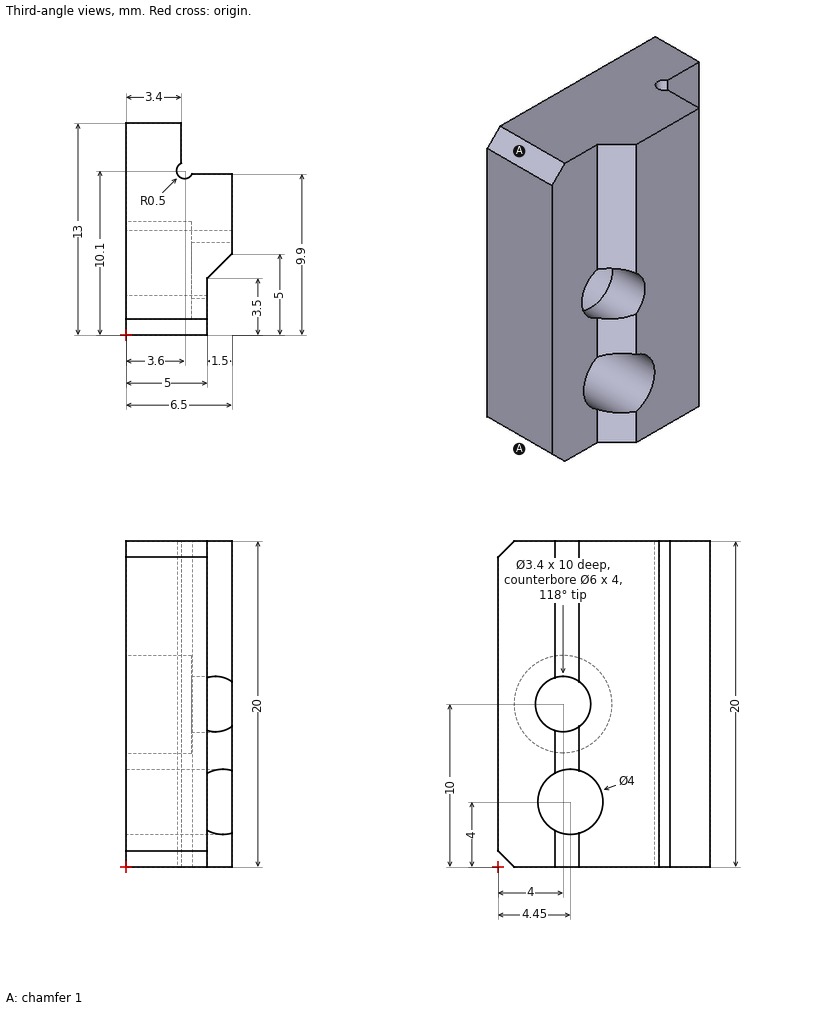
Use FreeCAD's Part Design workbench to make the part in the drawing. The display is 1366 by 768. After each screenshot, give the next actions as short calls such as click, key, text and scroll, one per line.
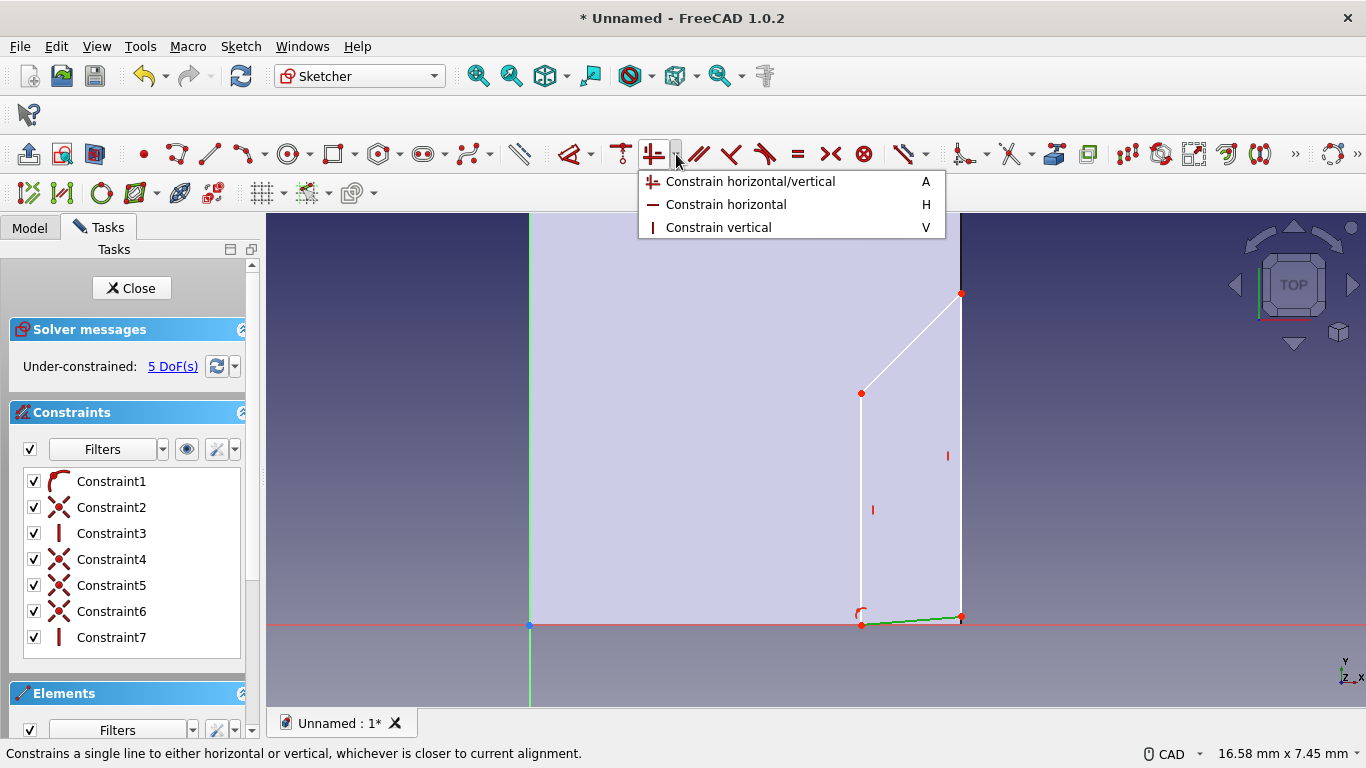
click(792, 204)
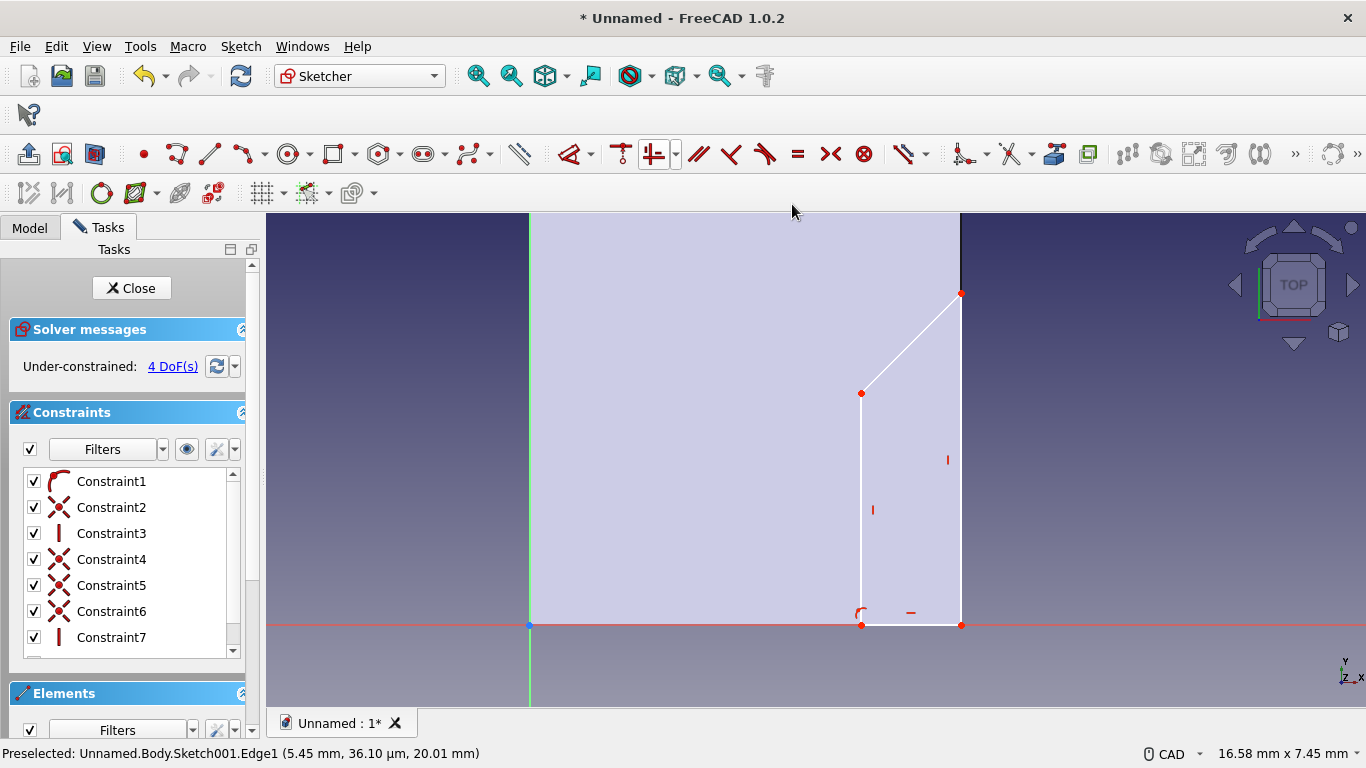
click(568, 154)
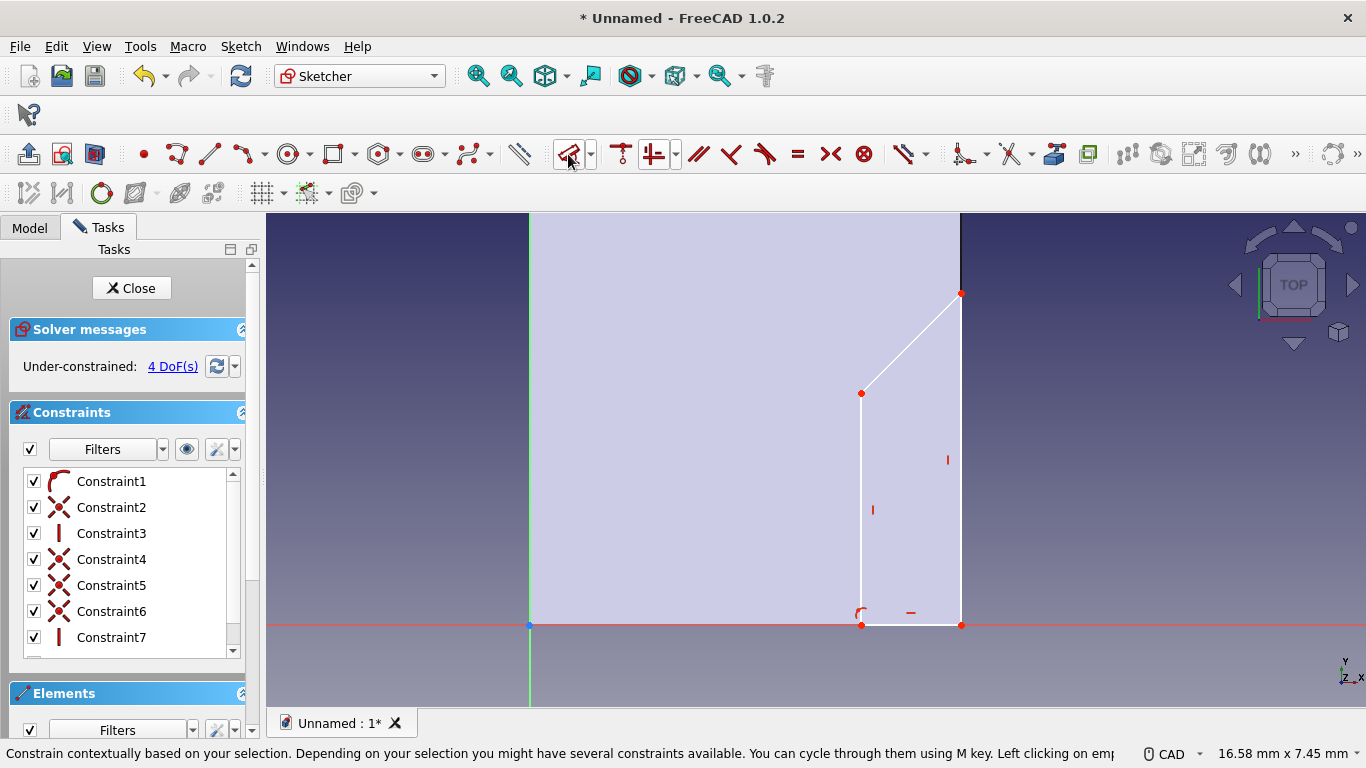
click(961, 526)
click(995, 460)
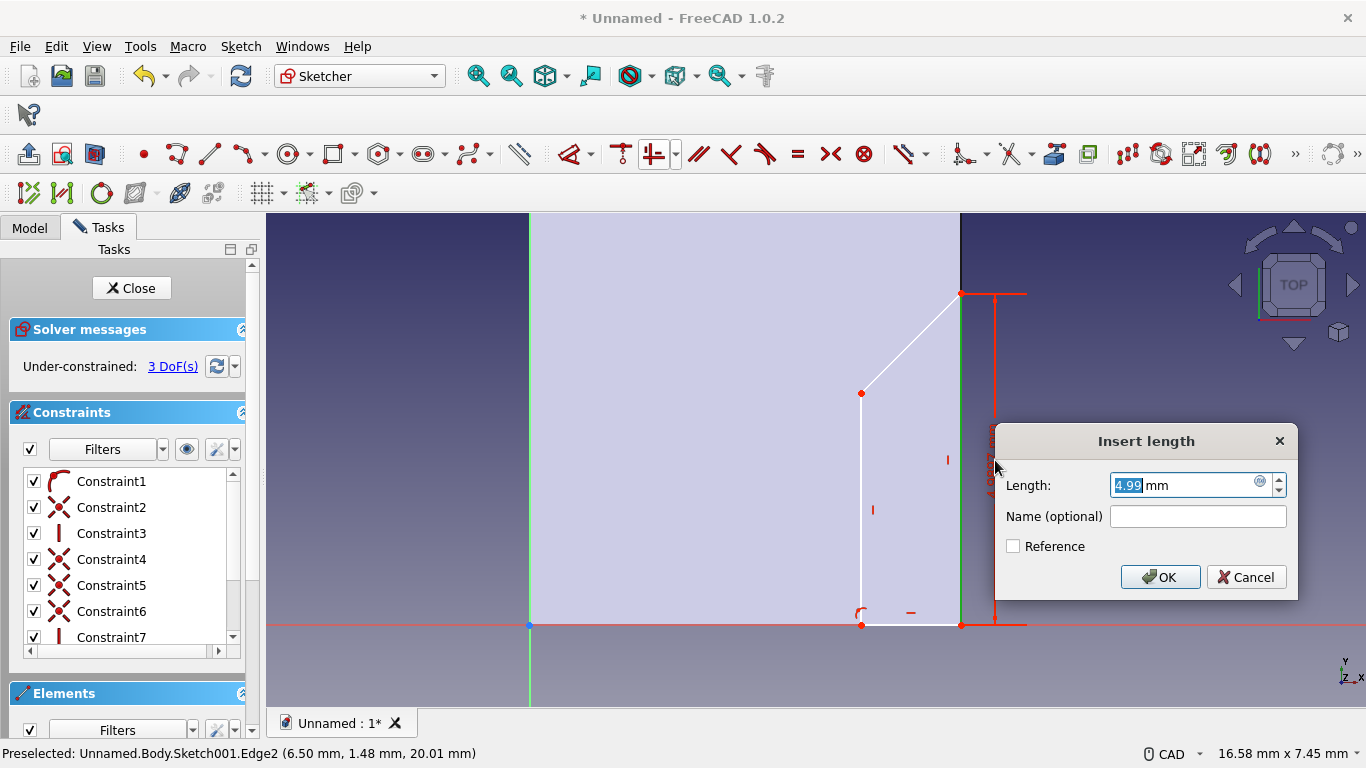
text(5)
key(Return)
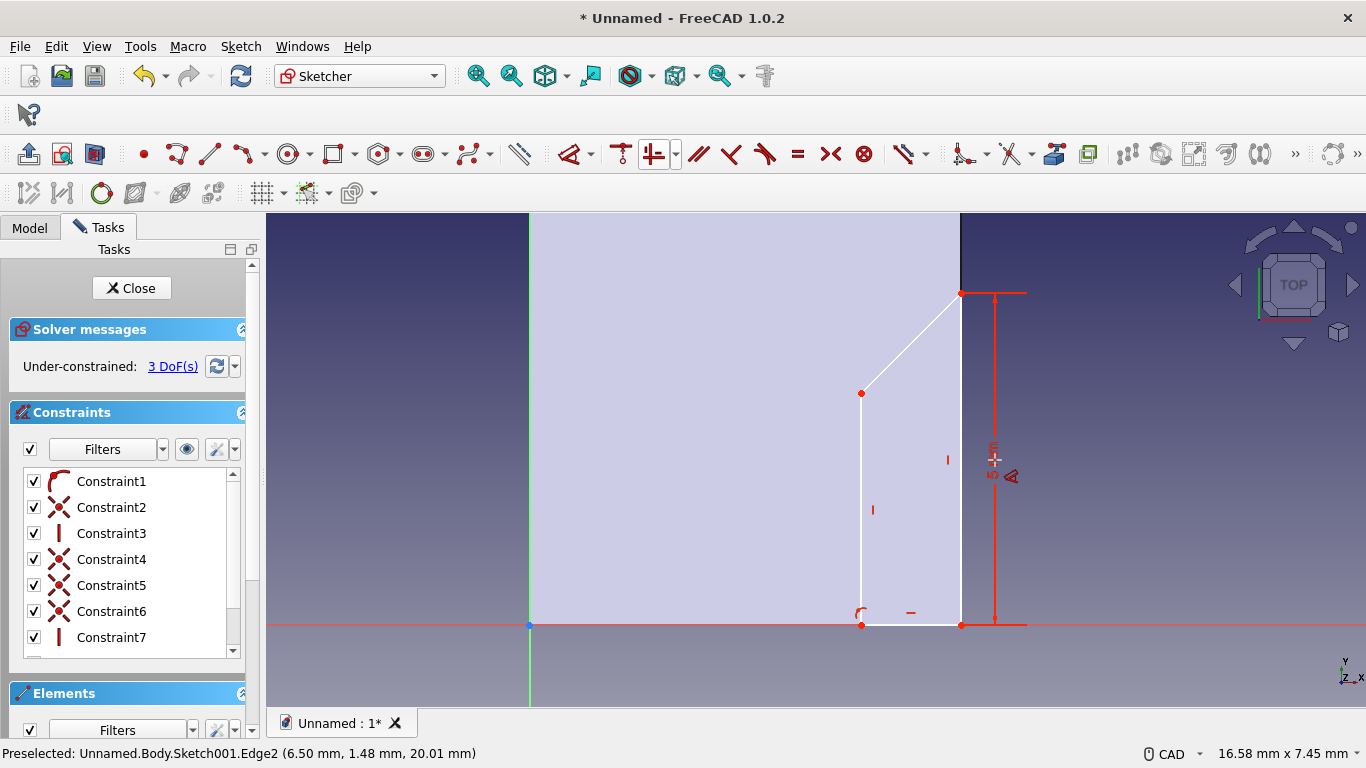
click(861, 625)
click(695, 659)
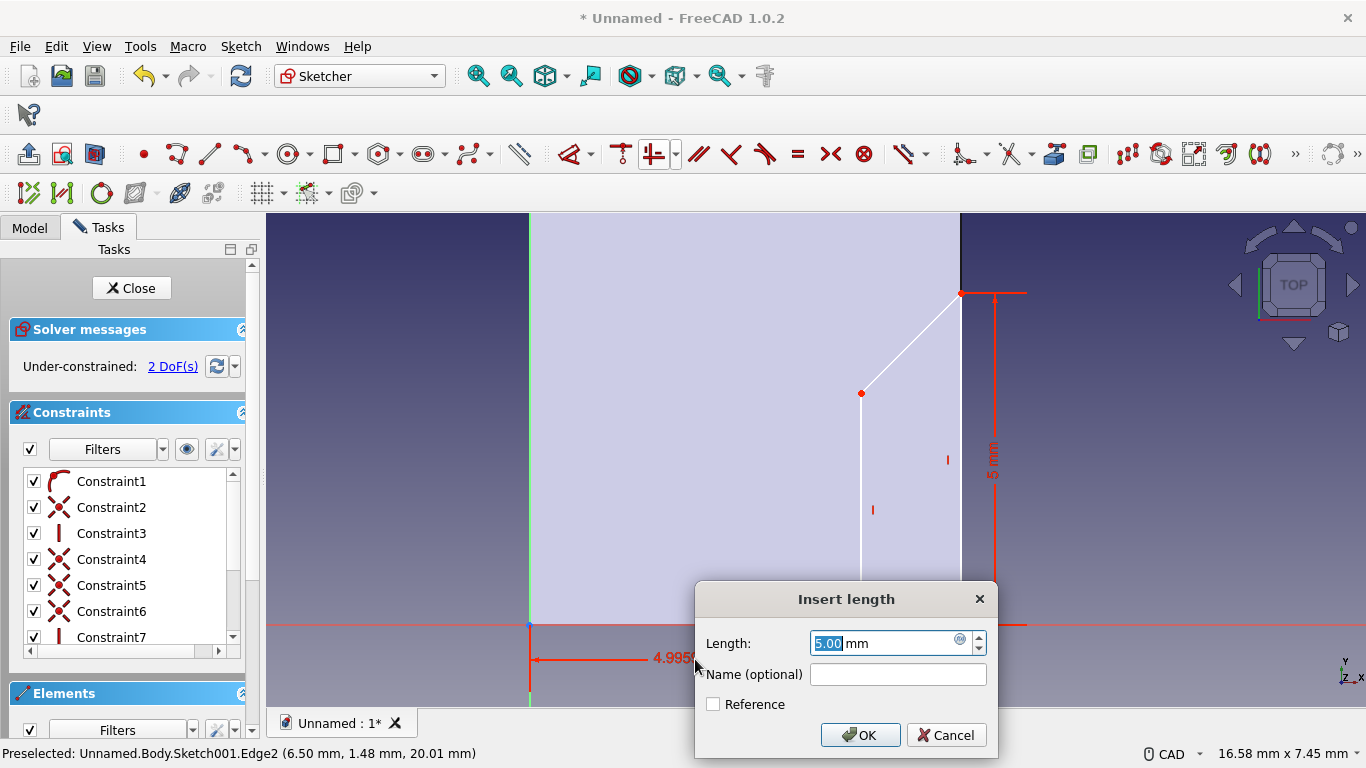
text(5)
key(Return)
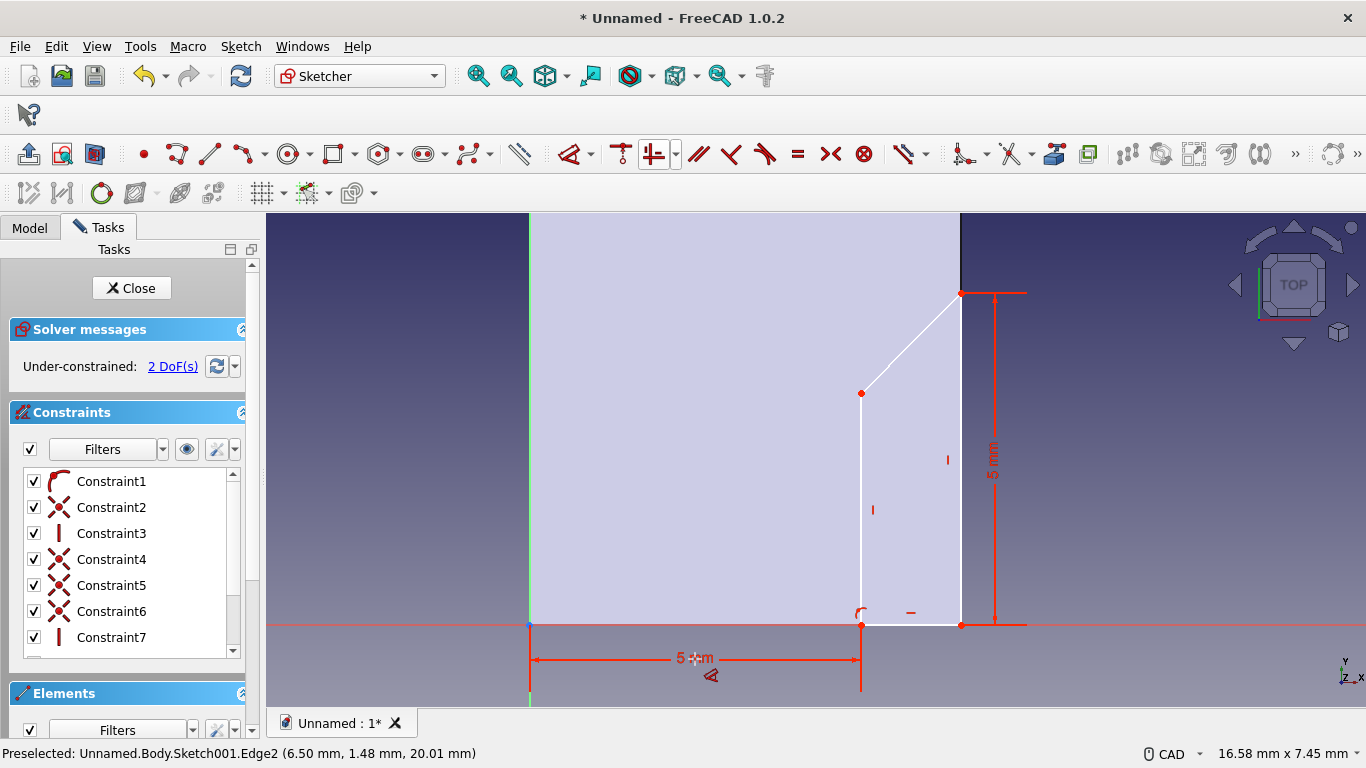
click(891, 625)
click(911, 659)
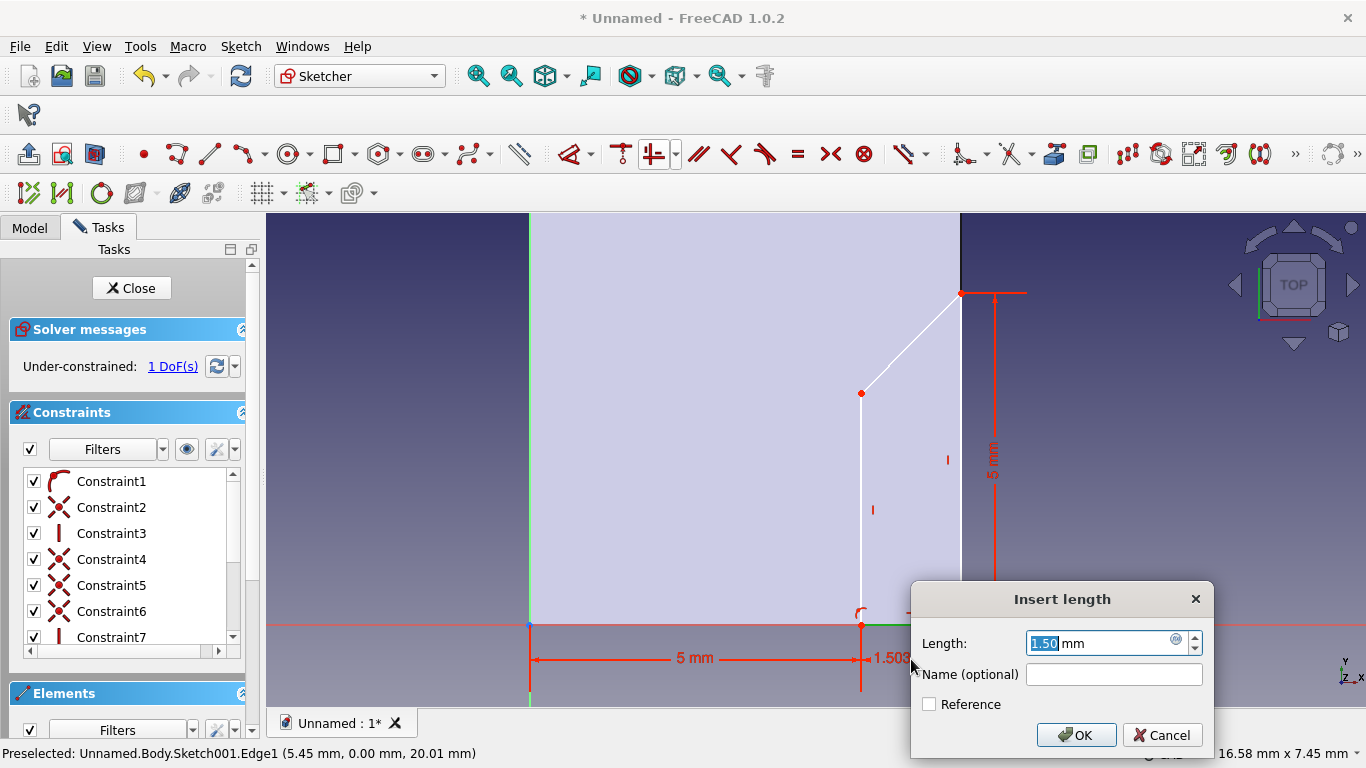
text(1.5)
key(Return)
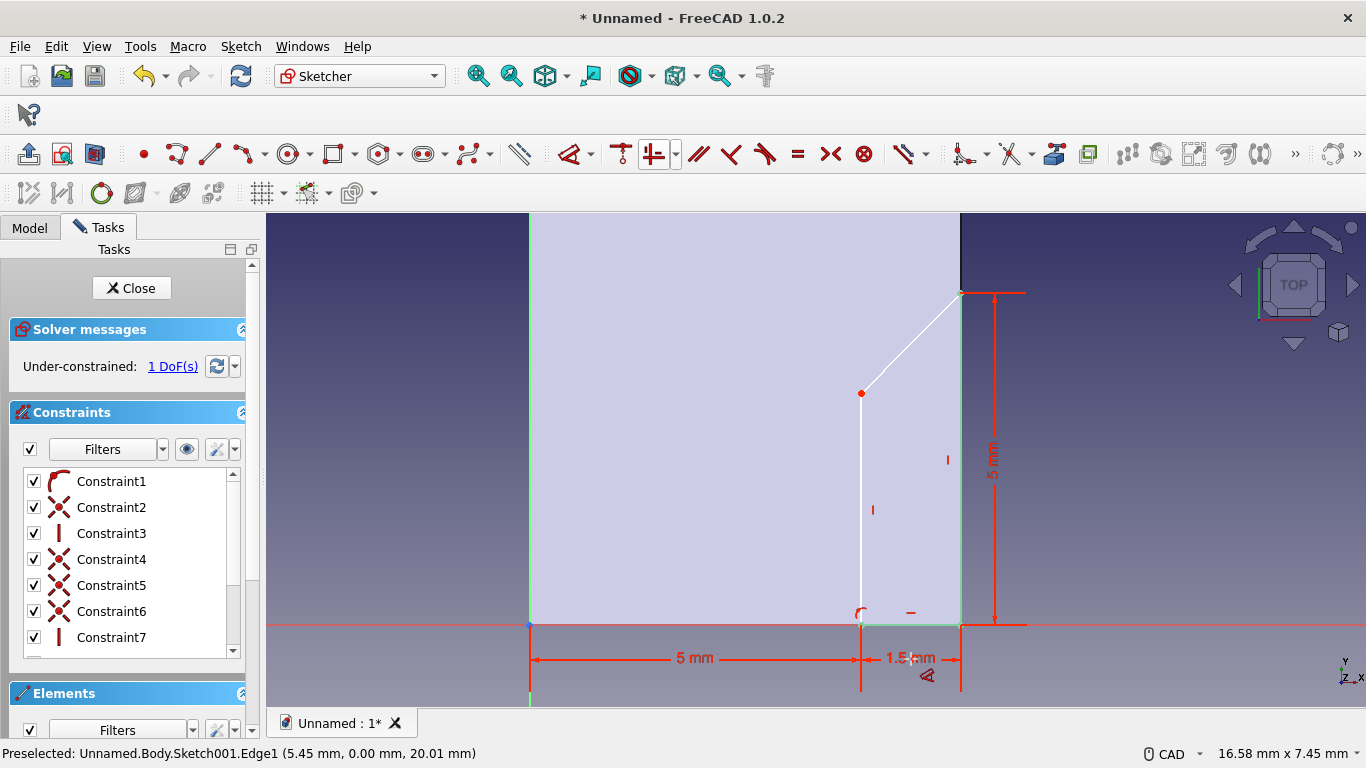
click(861, 463)
click(895, 510)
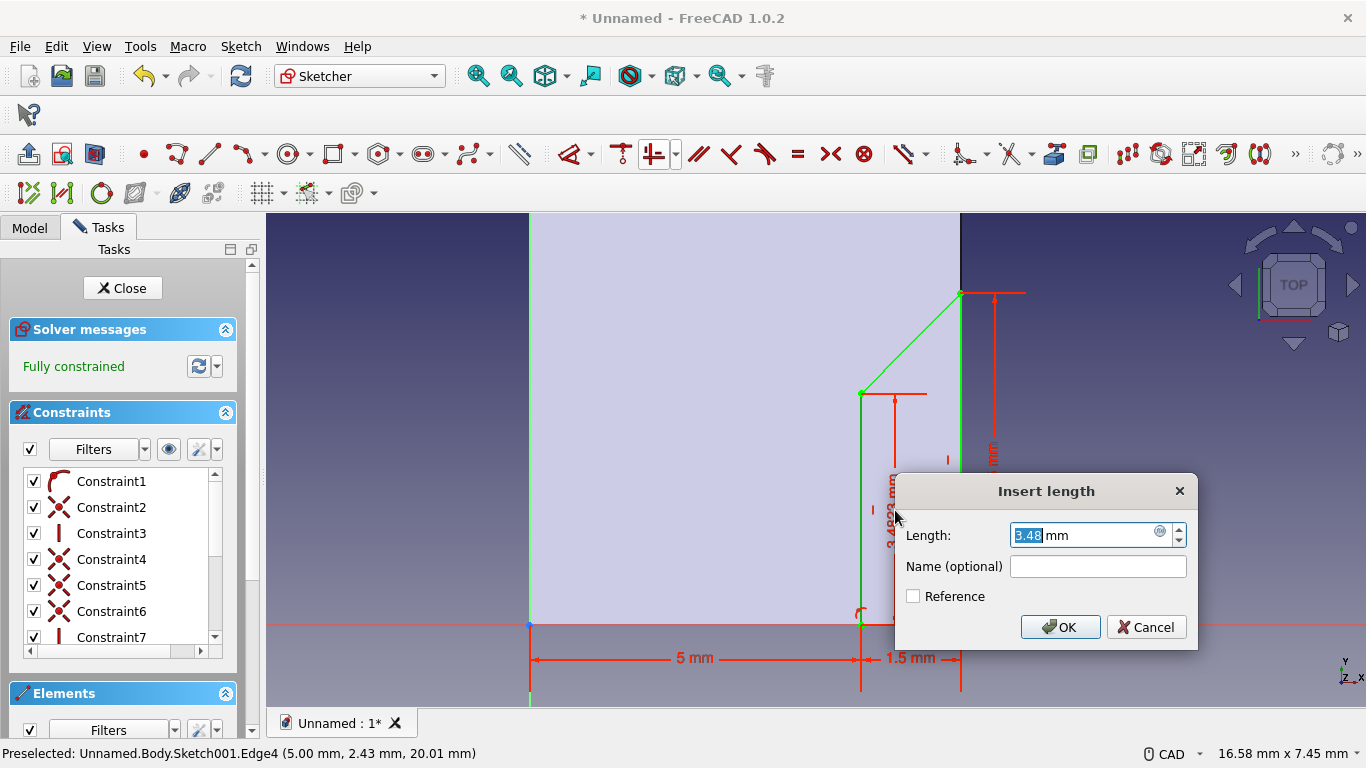
text(3.5)
key(Return)
key(Escape)